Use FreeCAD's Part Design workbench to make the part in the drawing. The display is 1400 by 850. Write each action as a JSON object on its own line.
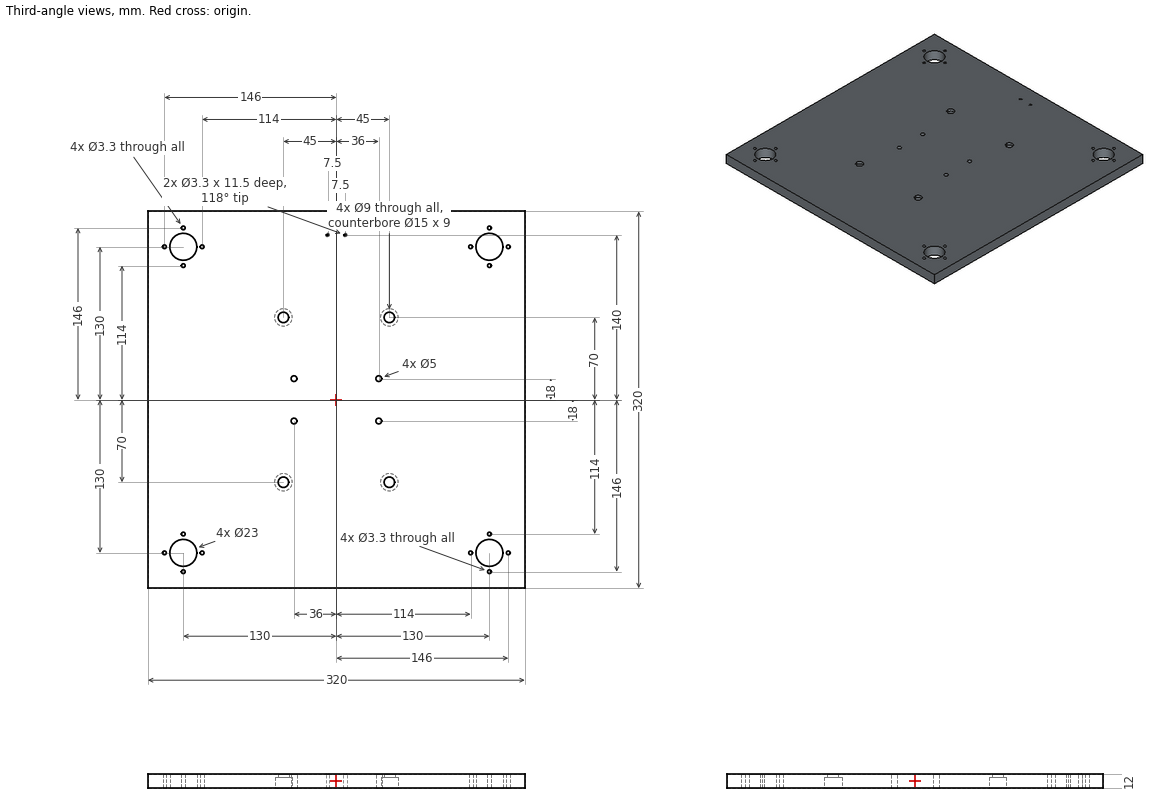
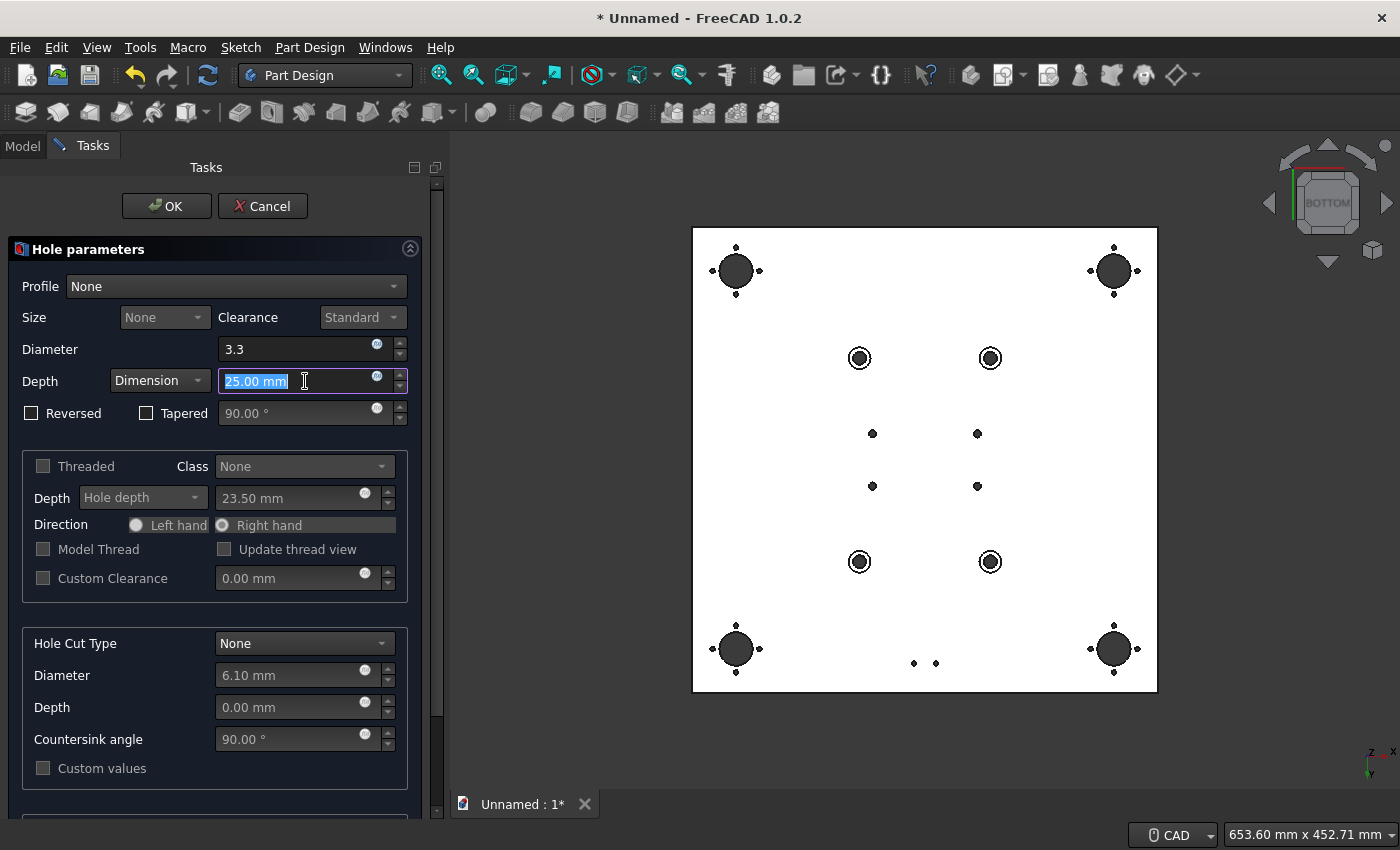
{"action": "type", "text": "11.5"}
{"action": "key", "text": "Tab"}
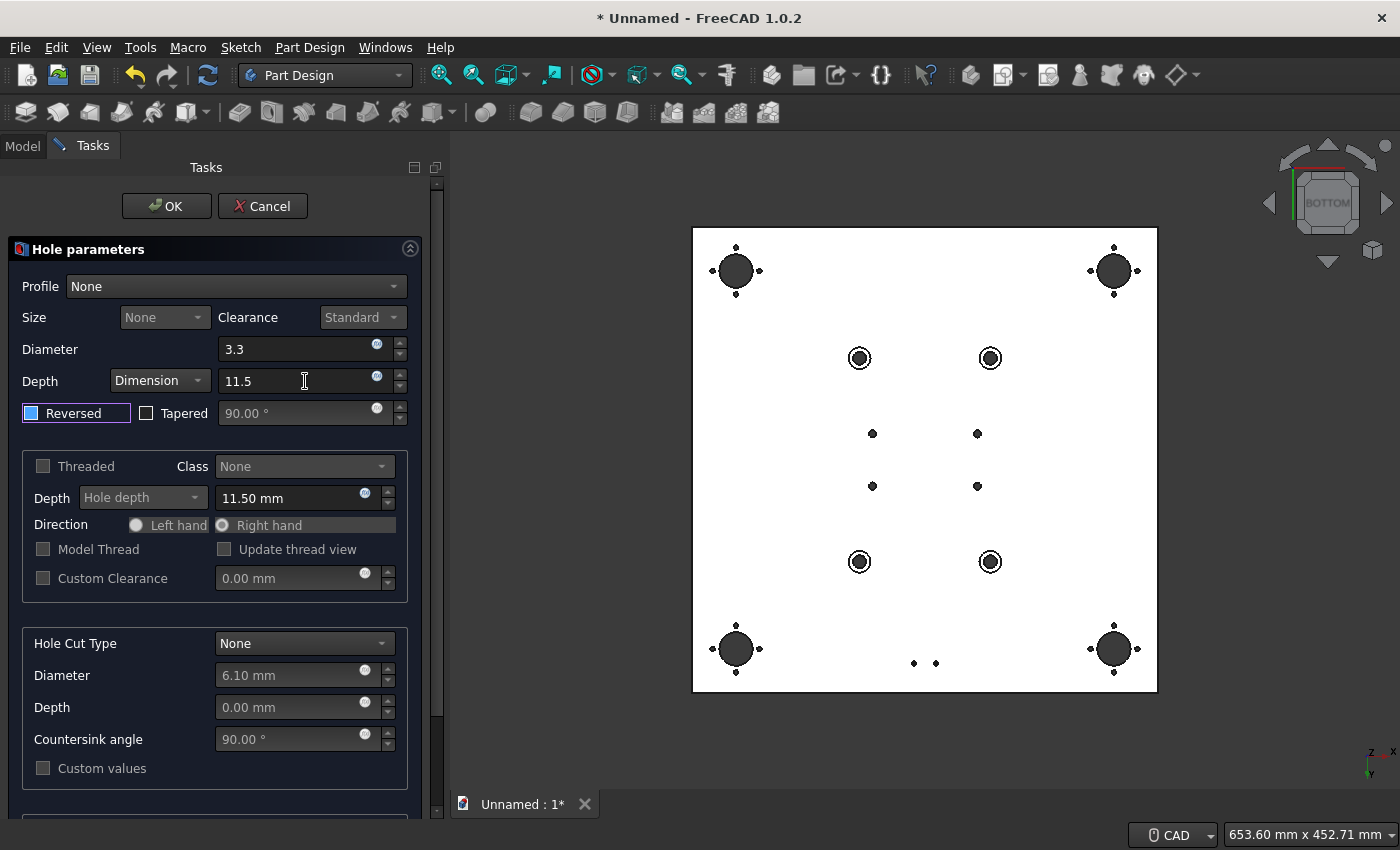
{"action": "left_click", "coordinate": [167, 206]}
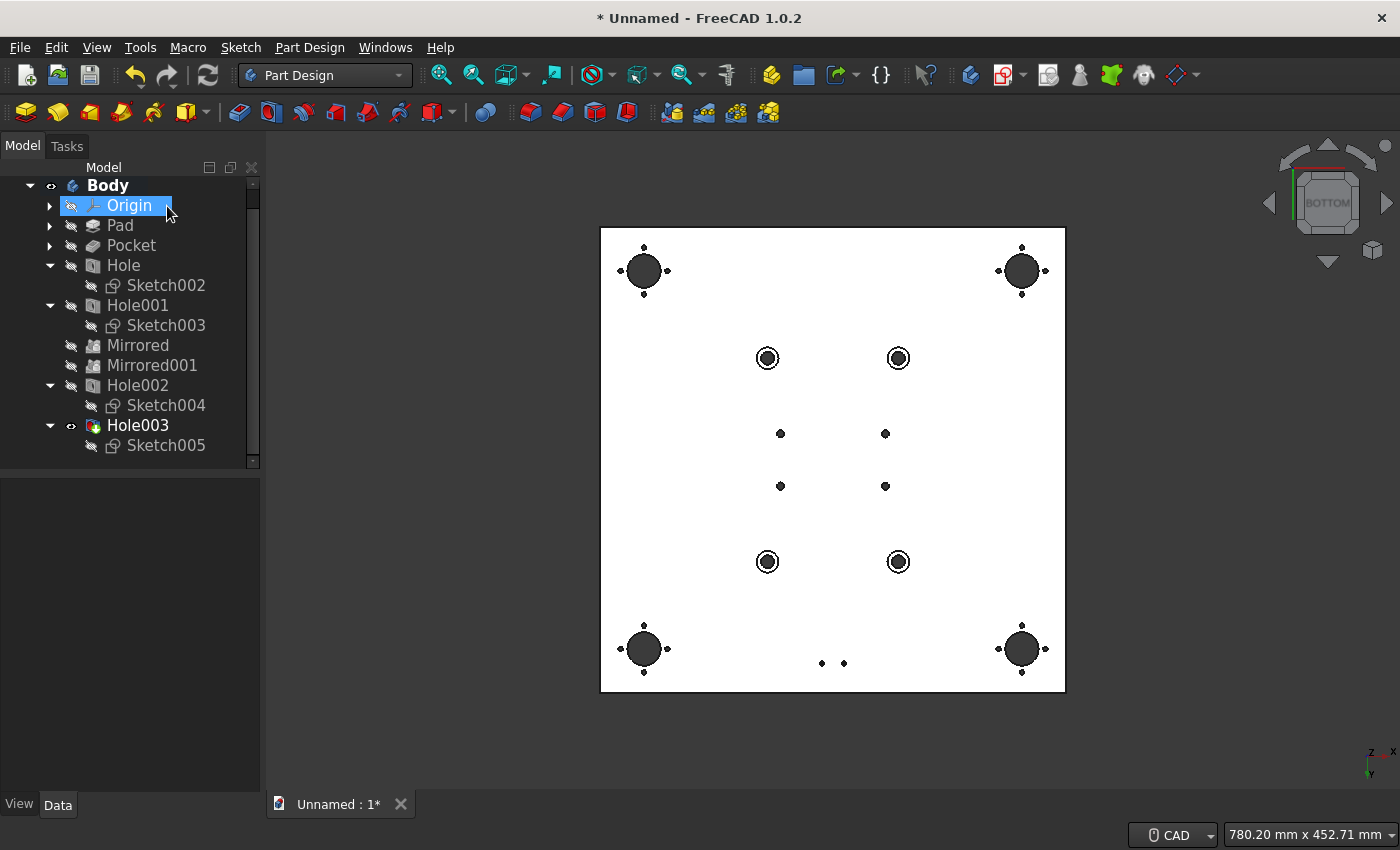
{"action": "key", "text": "0"}